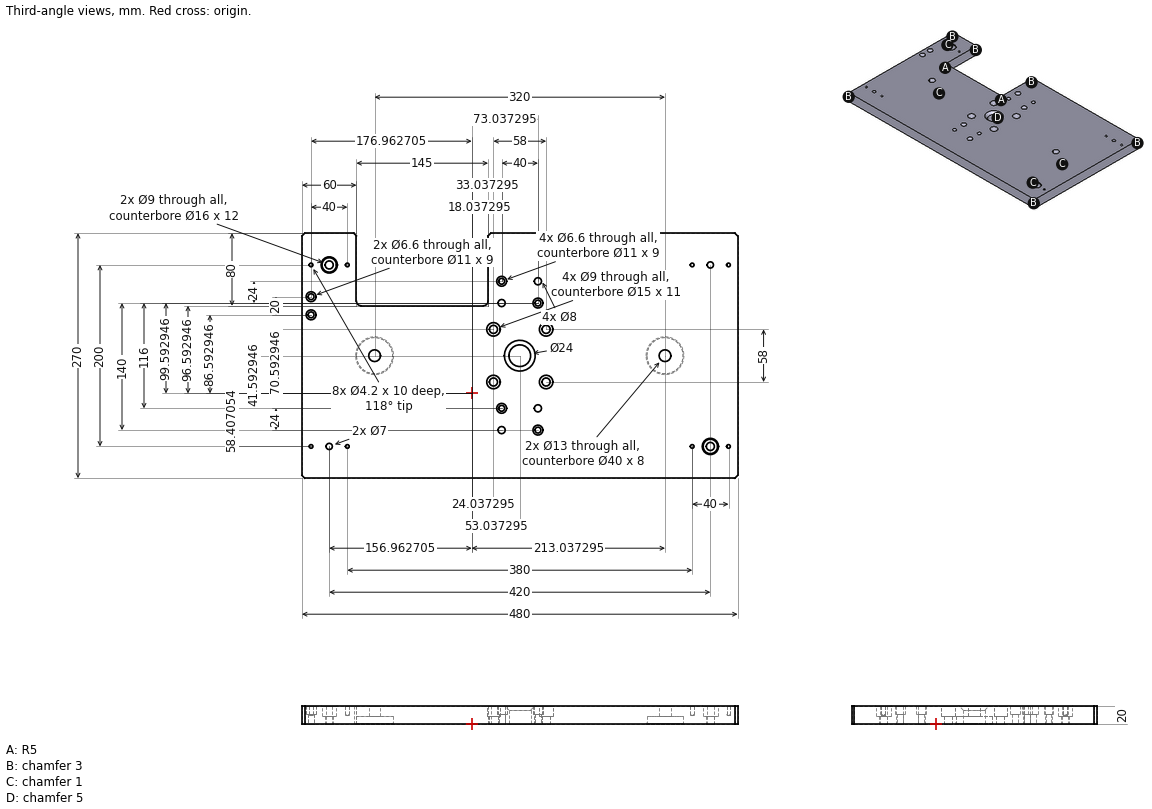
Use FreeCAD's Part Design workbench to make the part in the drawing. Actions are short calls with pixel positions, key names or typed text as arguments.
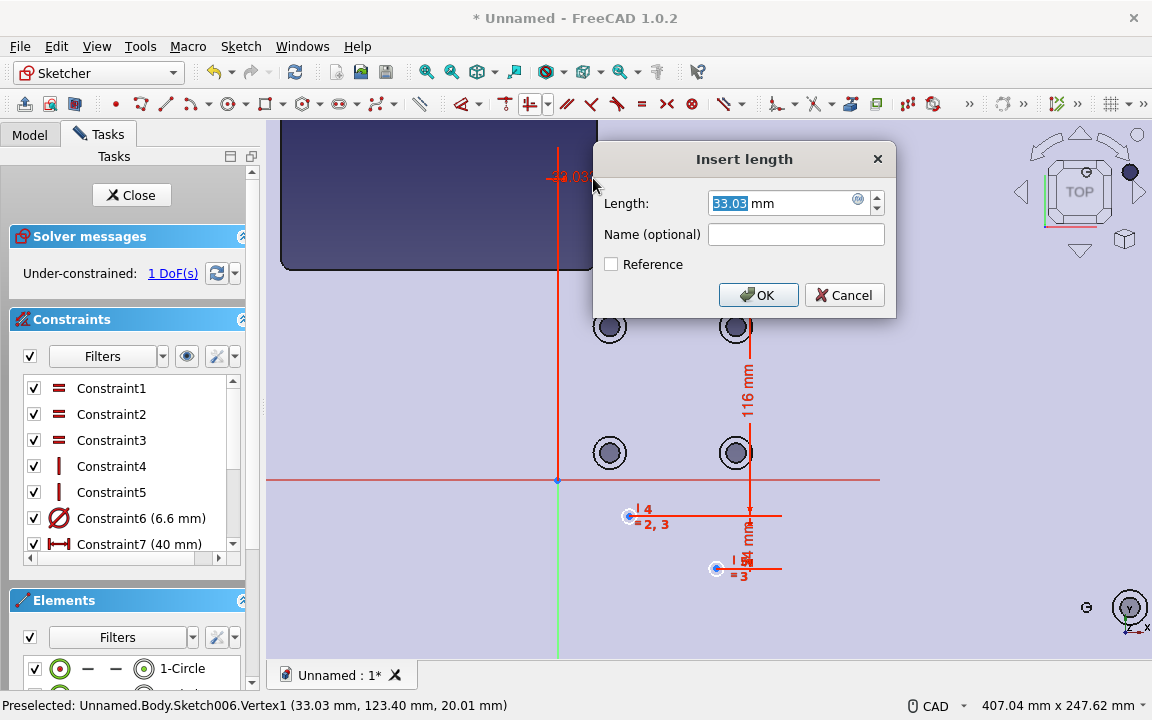
text(33.037295)
key(Return)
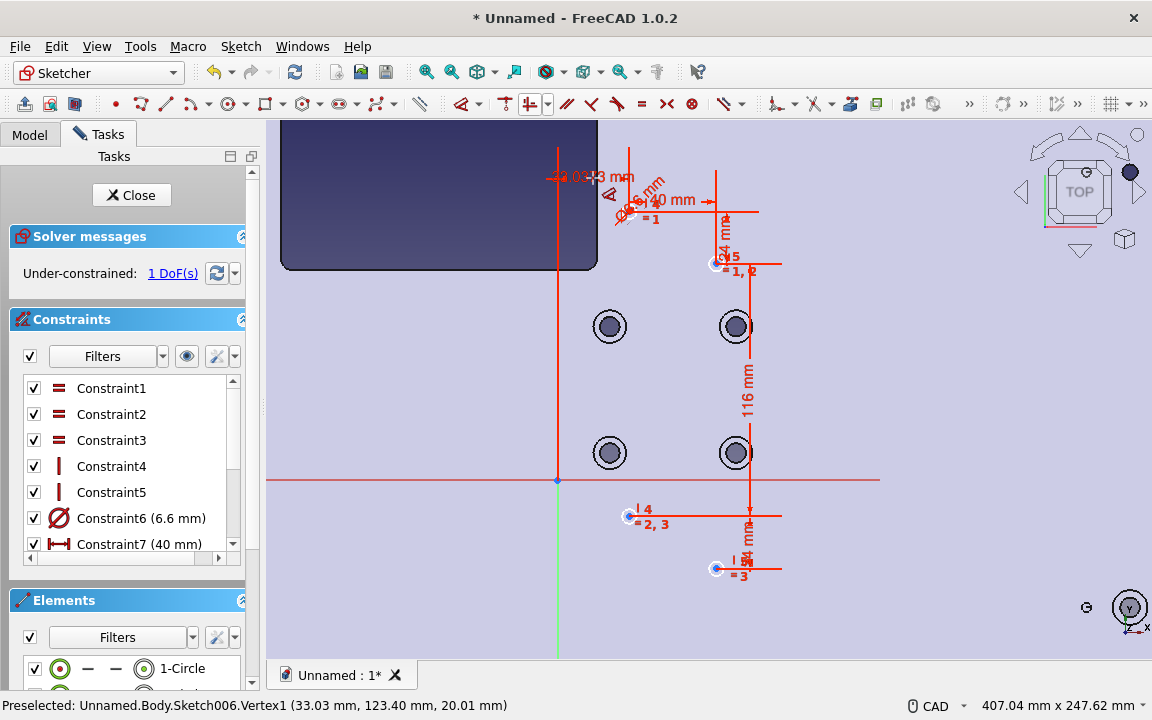
click(716, 264)
click(524, 372)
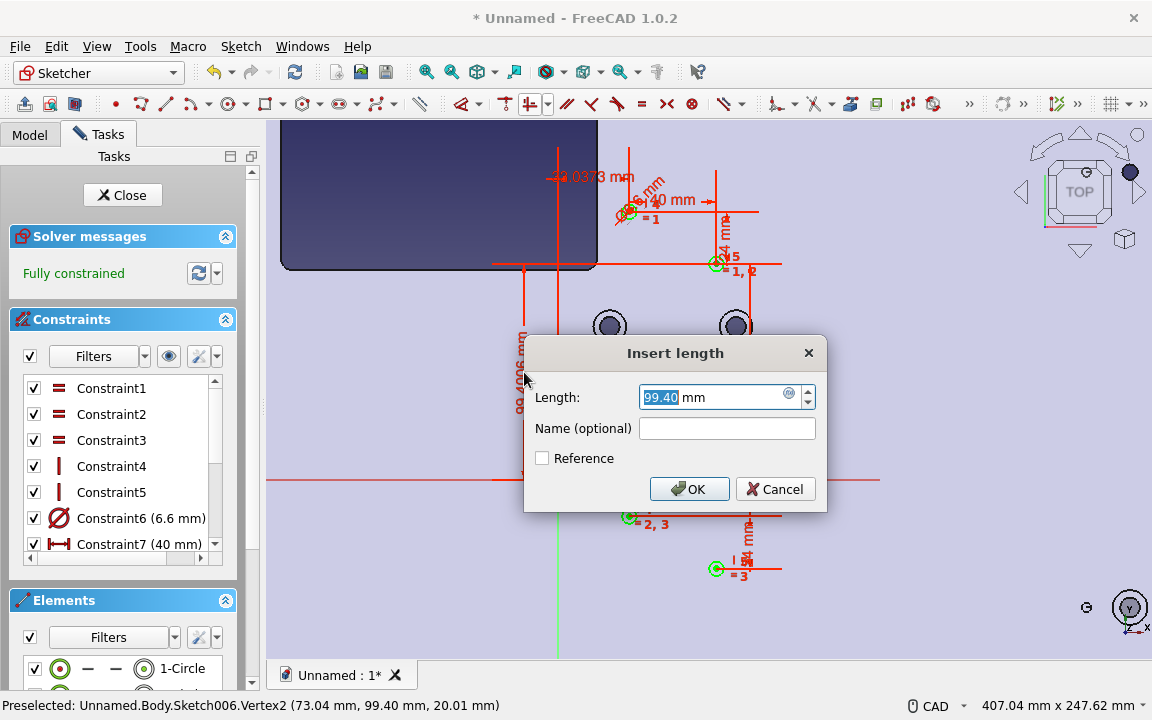
text(99.592946)
key(Return)
key(Escape)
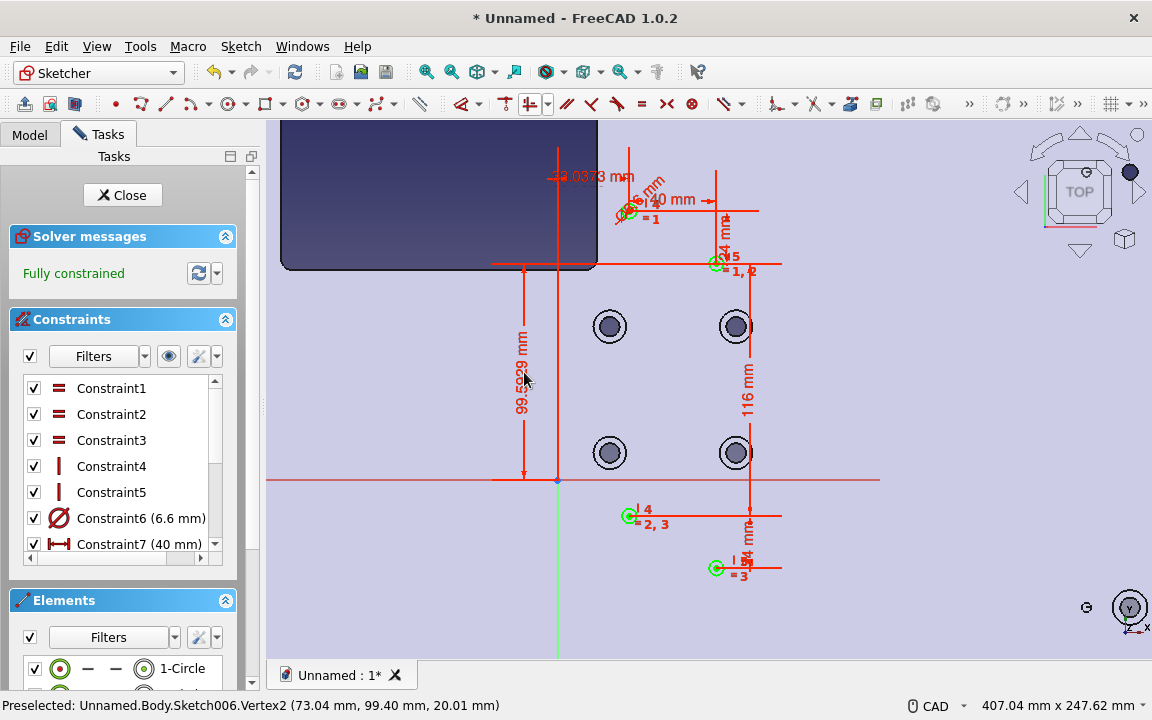
click(123, 195)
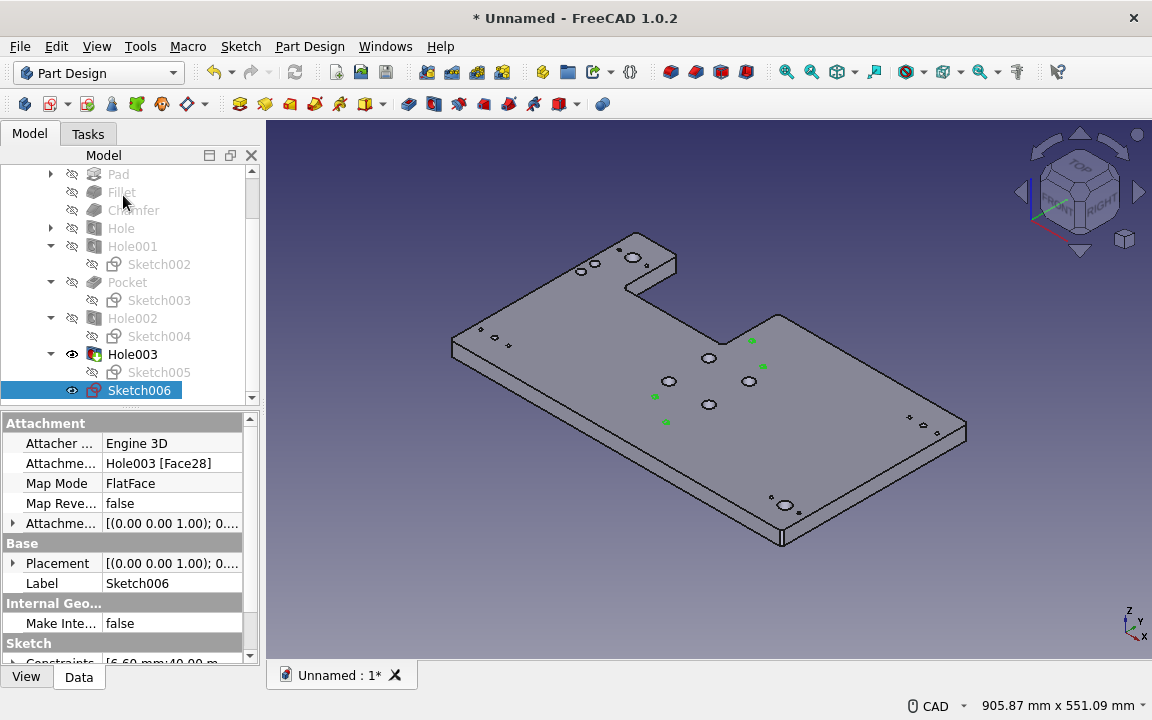
click(434, 104)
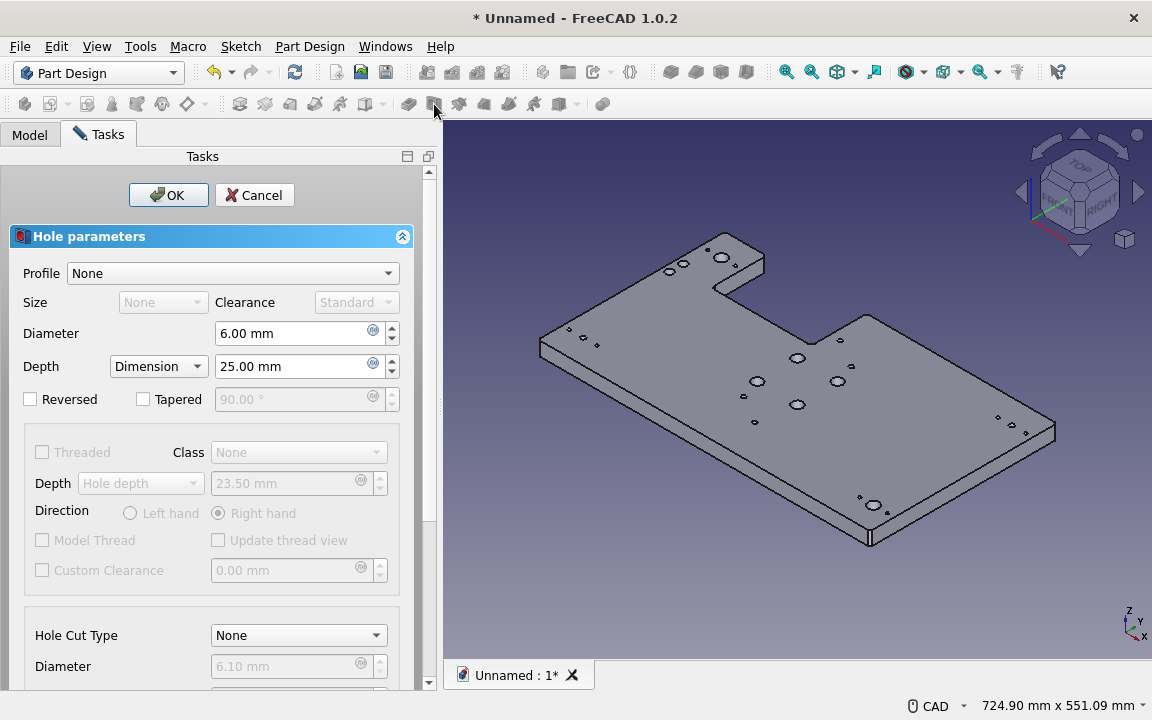
triple_click(300, 334)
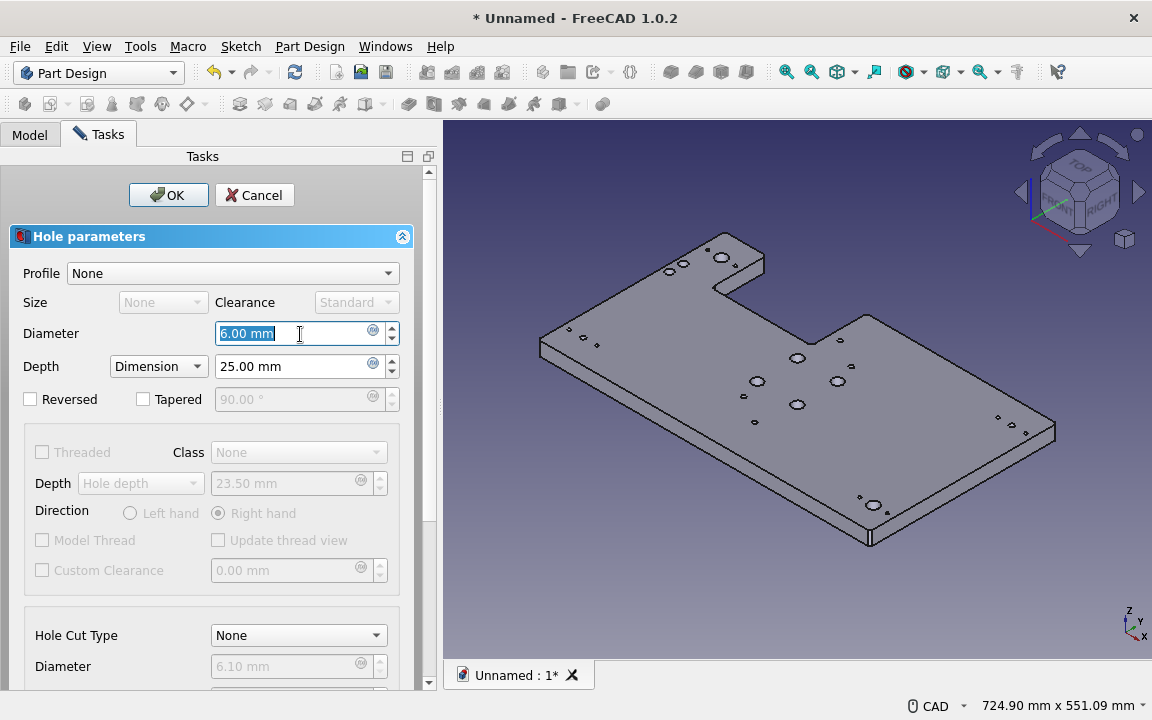
text(6.6)
key(Tab)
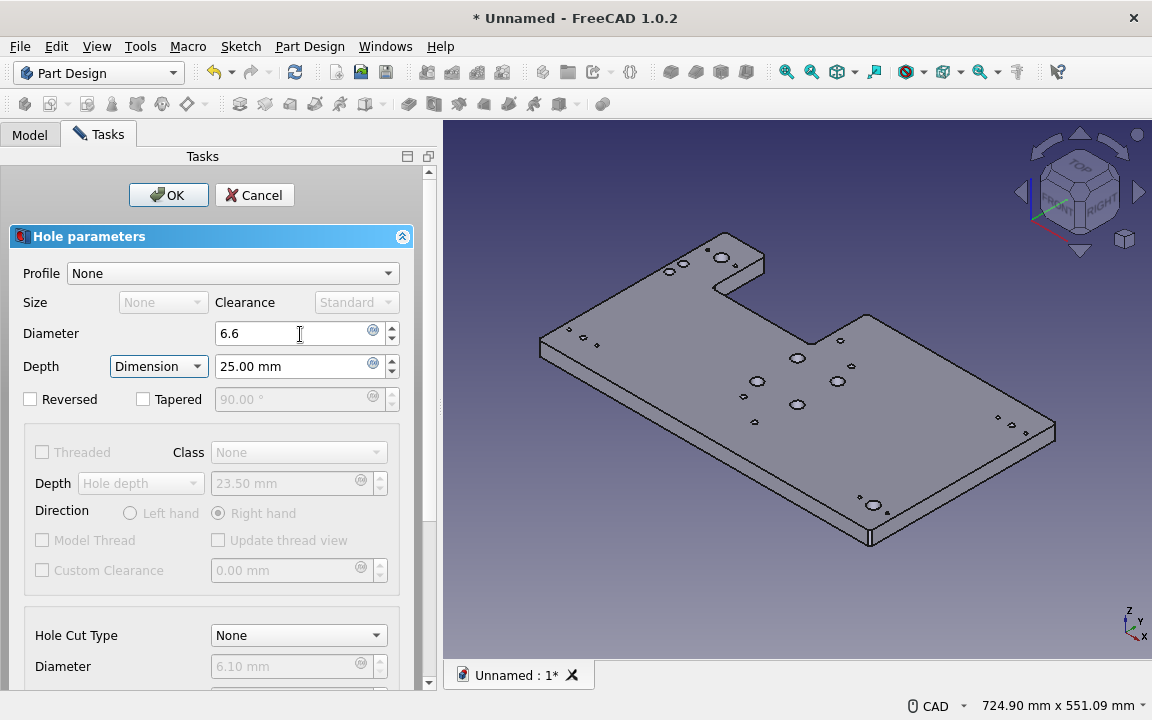
click(160, 366)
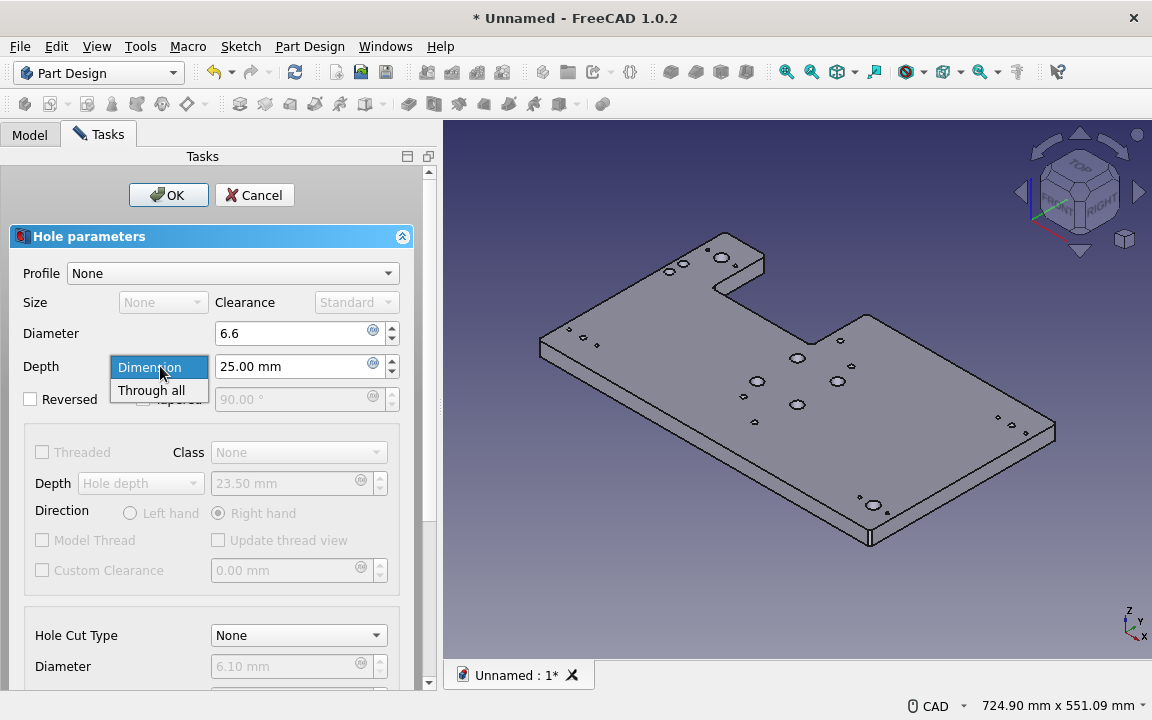
click(158, 390)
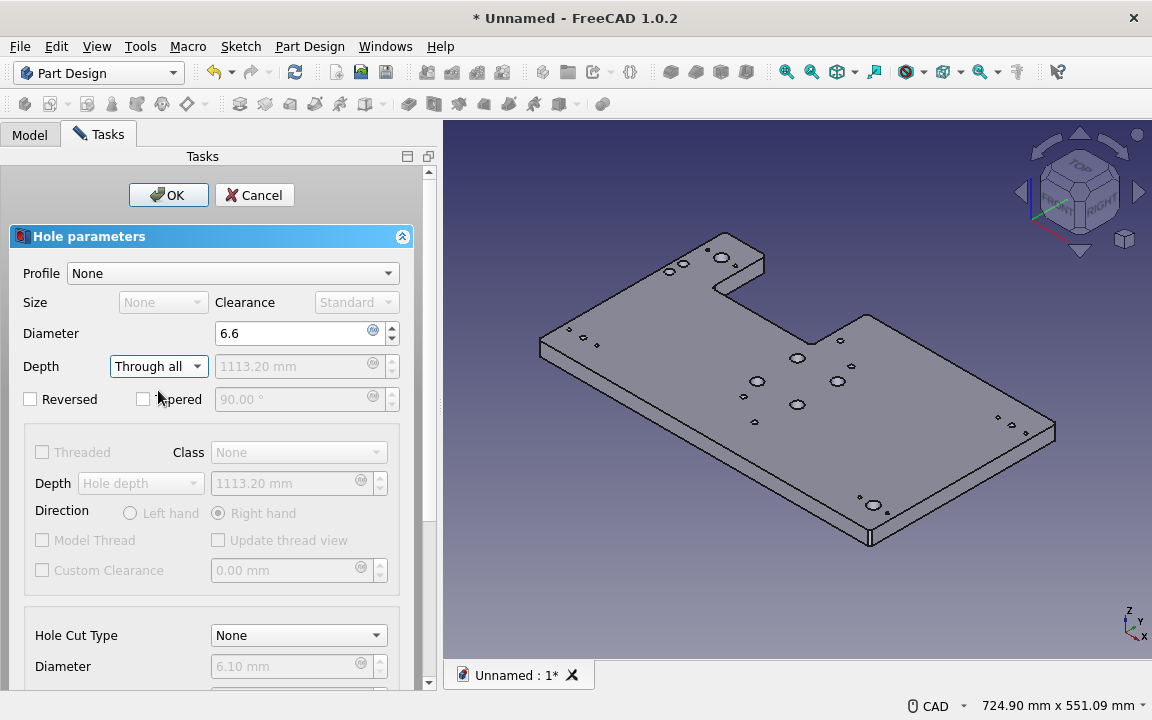
click(300, 636)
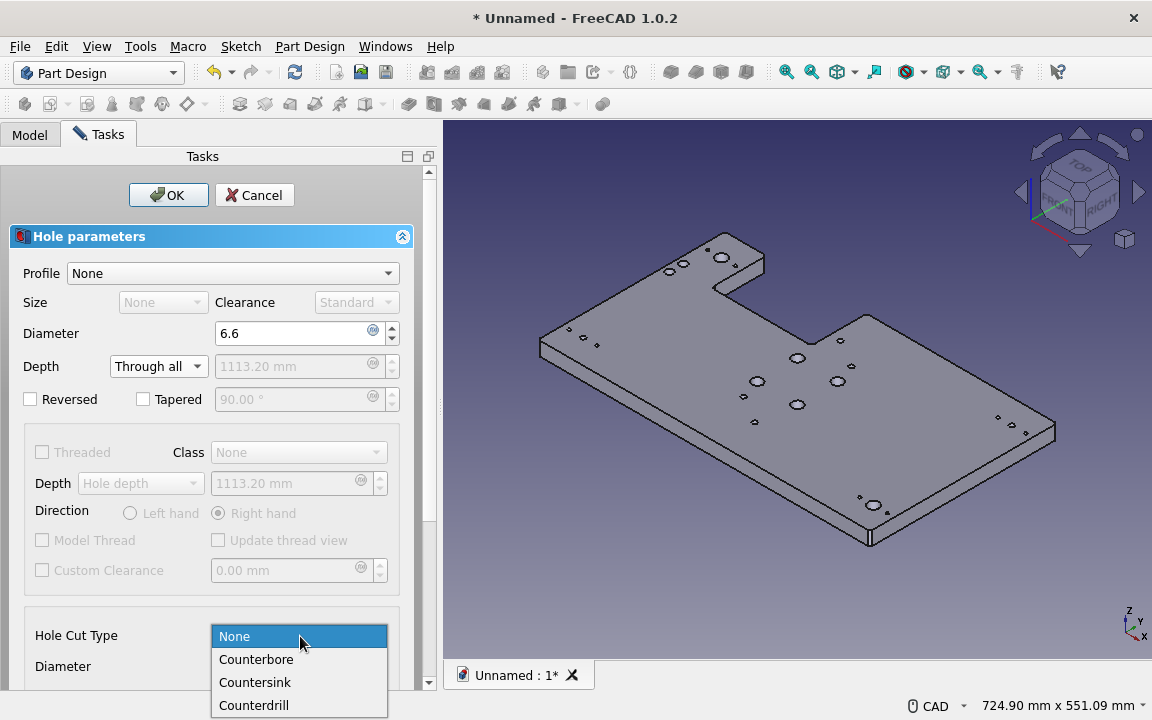
click(298, 660)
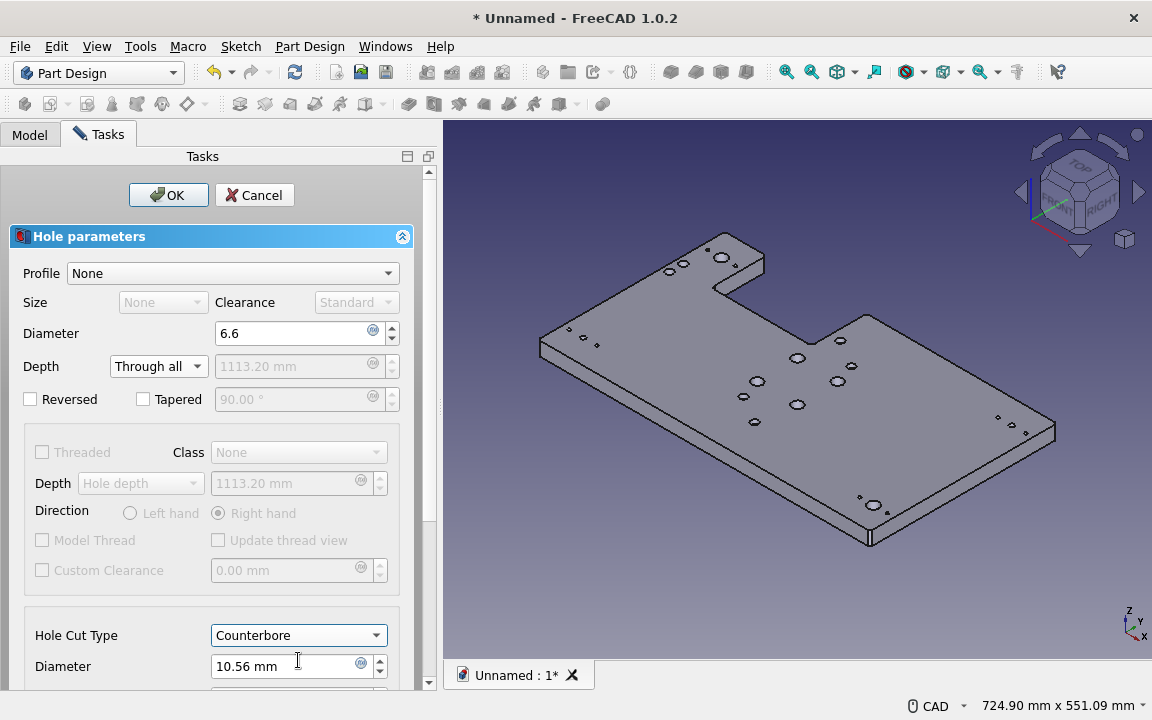
triple_click(292, 666)